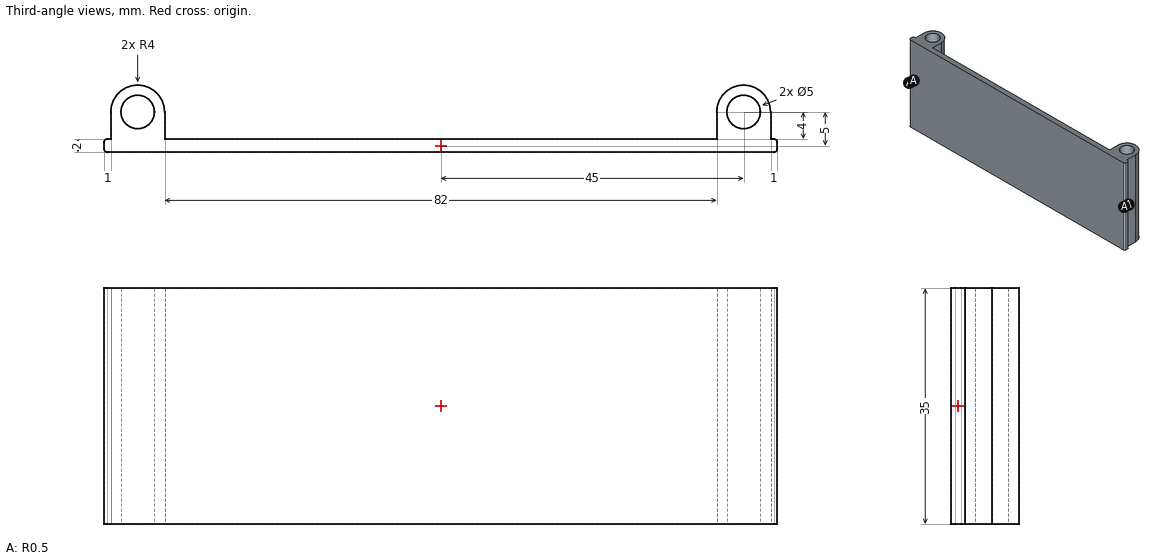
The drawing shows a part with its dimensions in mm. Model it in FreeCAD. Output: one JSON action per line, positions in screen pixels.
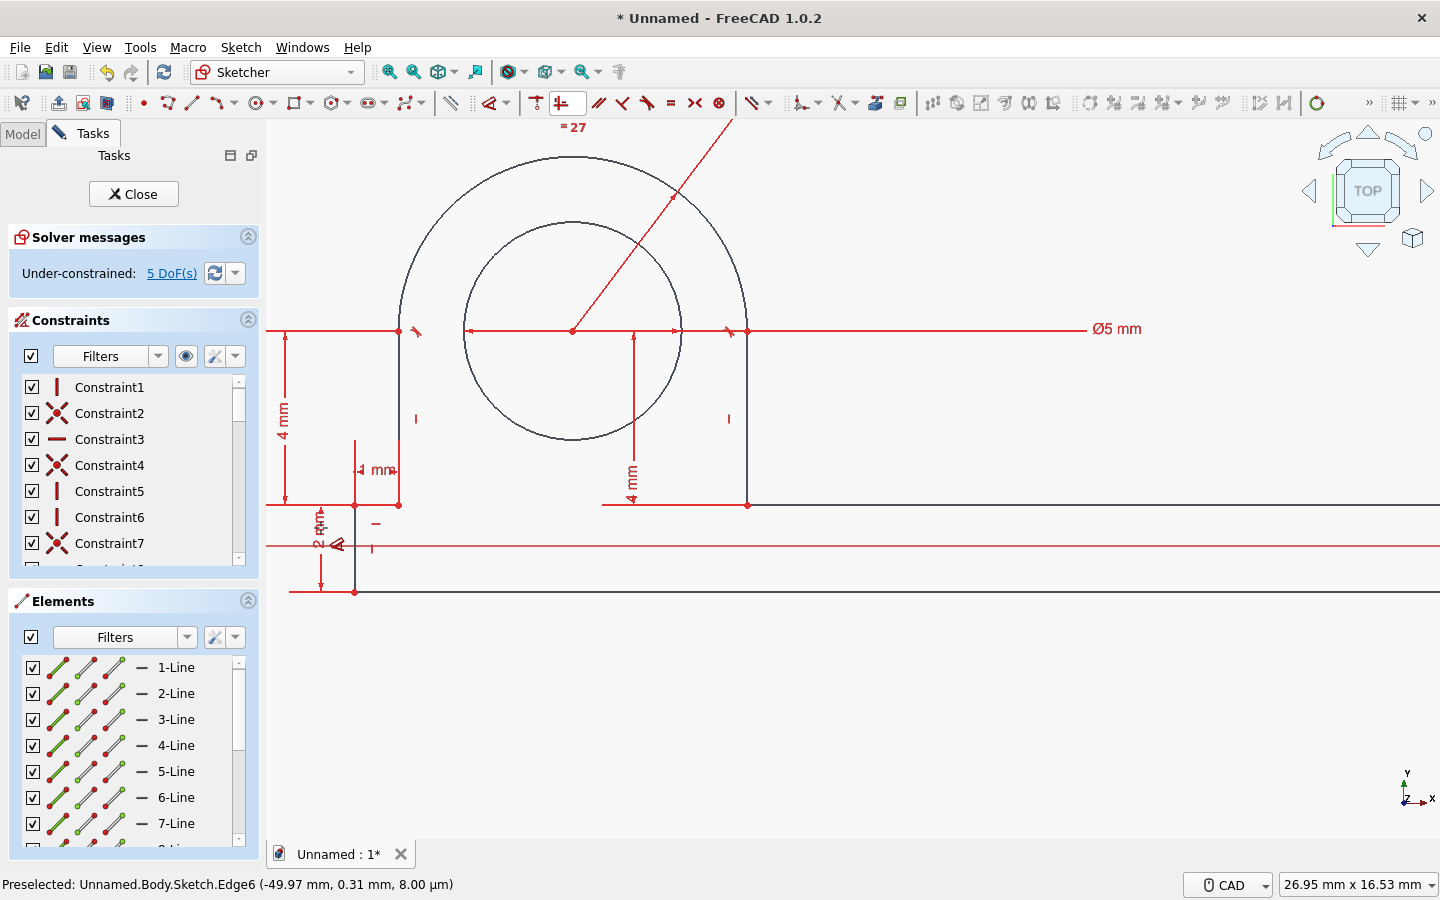
{"action": "scroll", "coordinate": [438, 500], "scroll_direction": "down", "scroll_amount": 9}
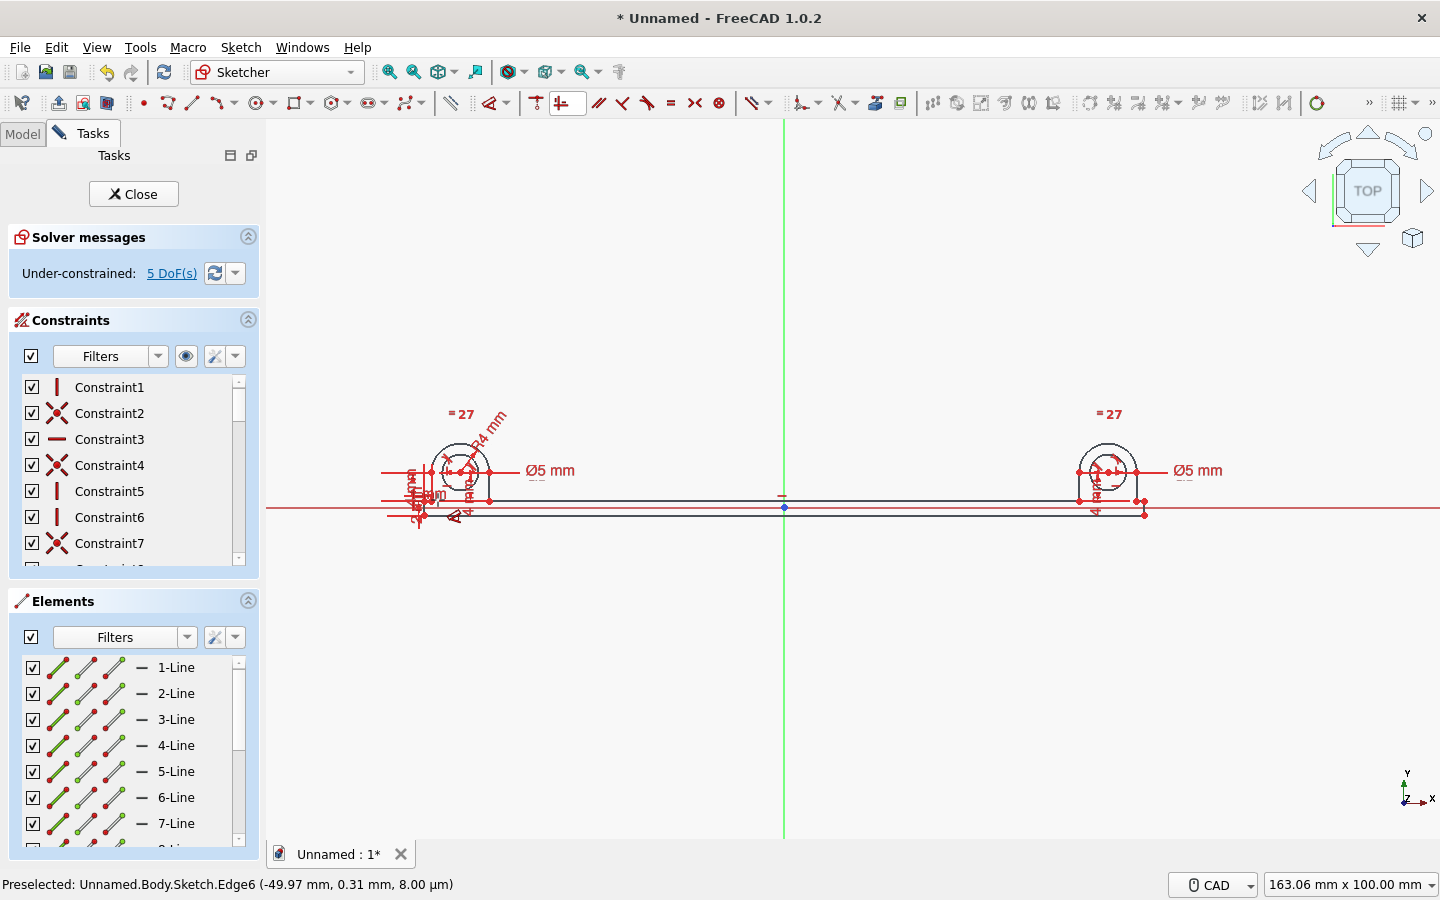
{"action": "scroll", "coordinate": [1144, 511], "scroll_direction": "up", "scroll_amount": 8}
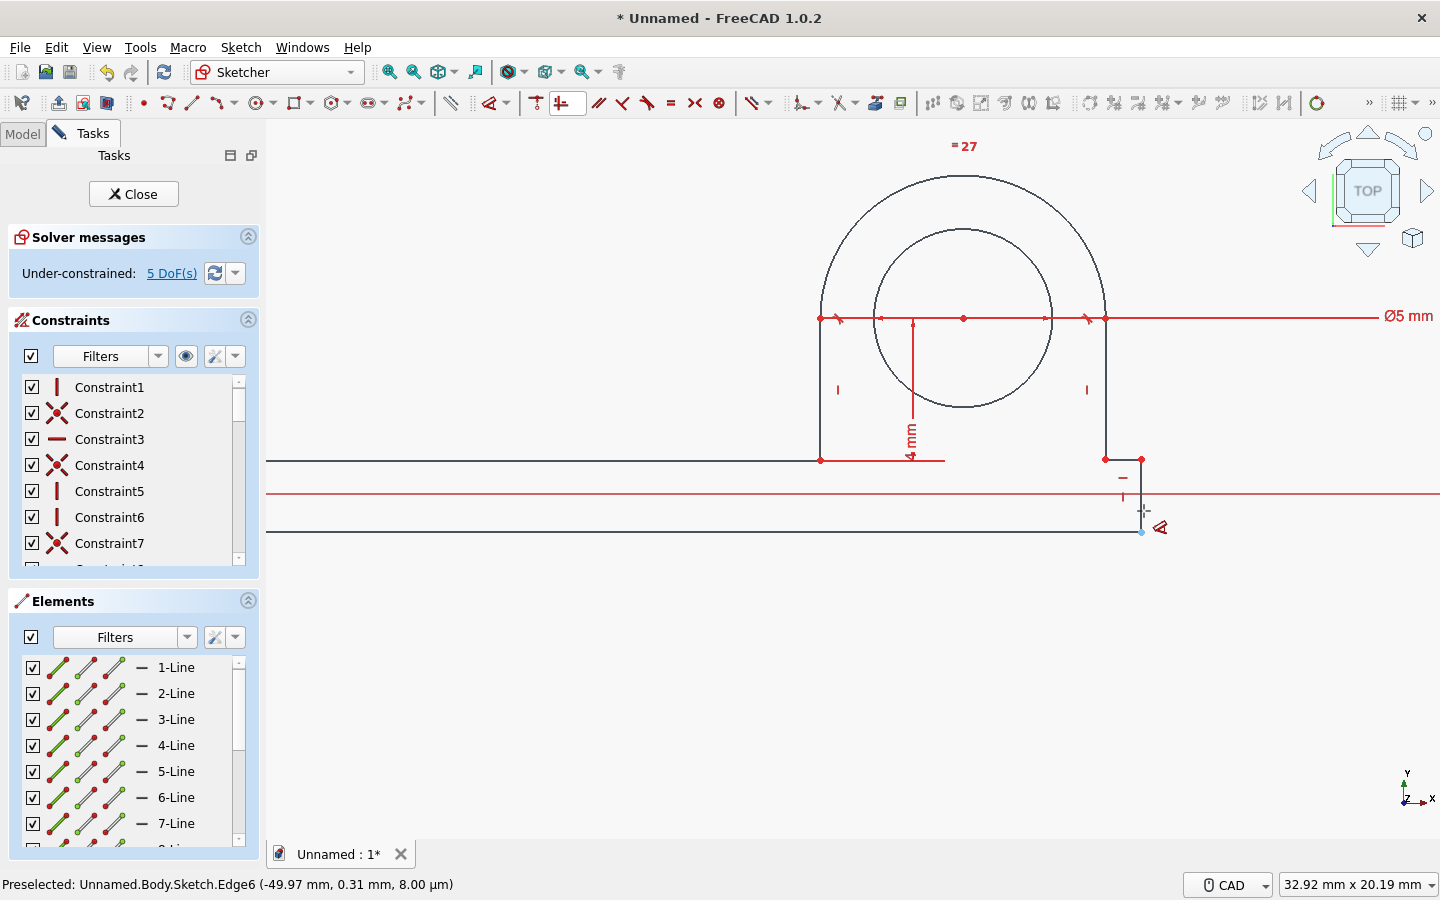
{"action": "left_click", "coordinate": [1141, 511]}
{"action": "left_click", "coordinate": [1175, 479]}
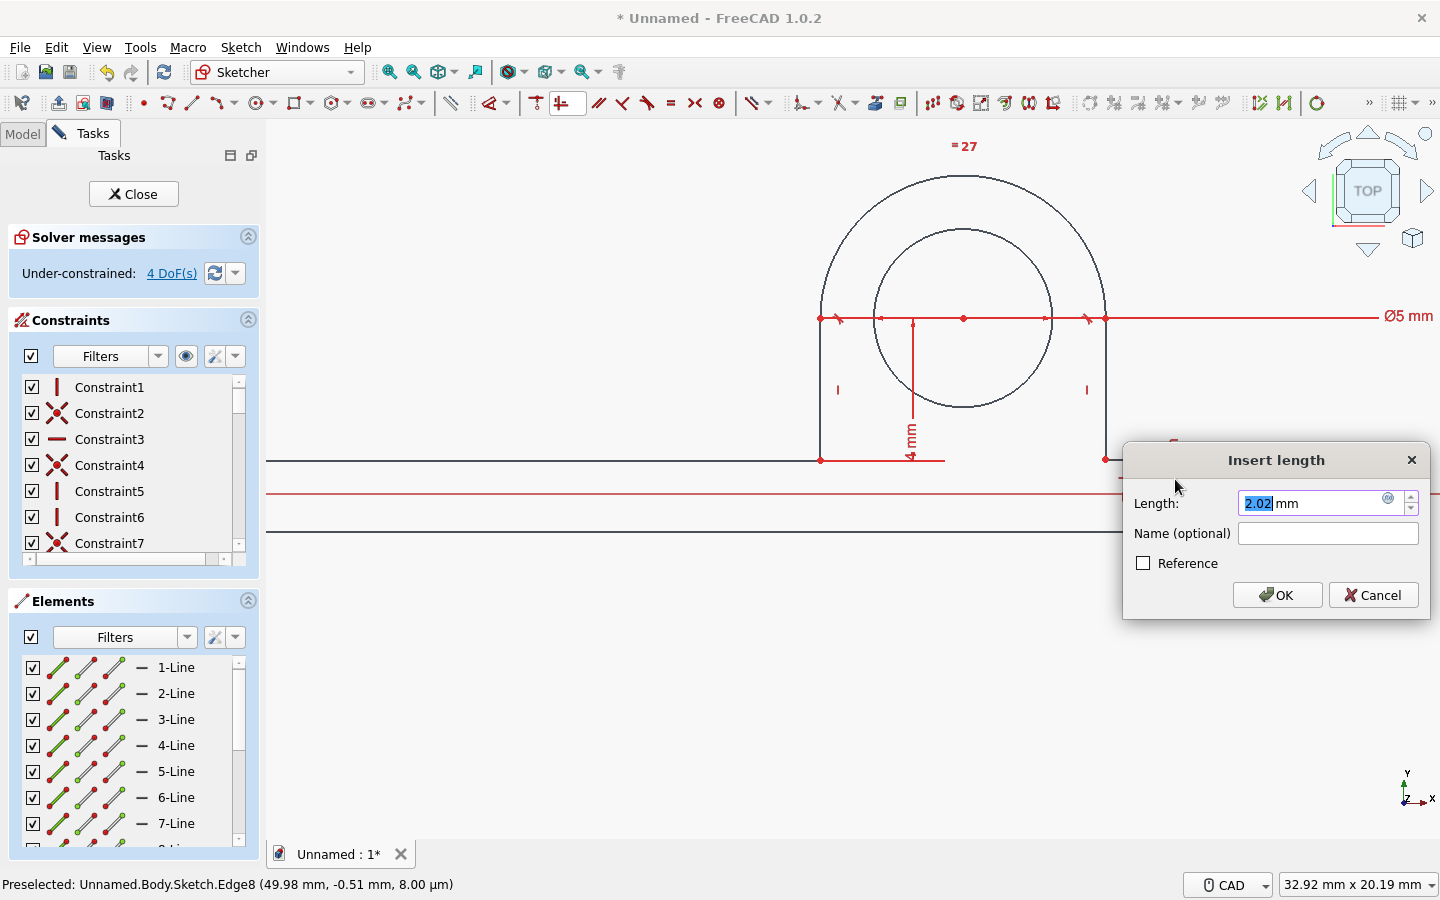
{"action": "type", "text": "2"}
{"action": "key", "text": "Return"}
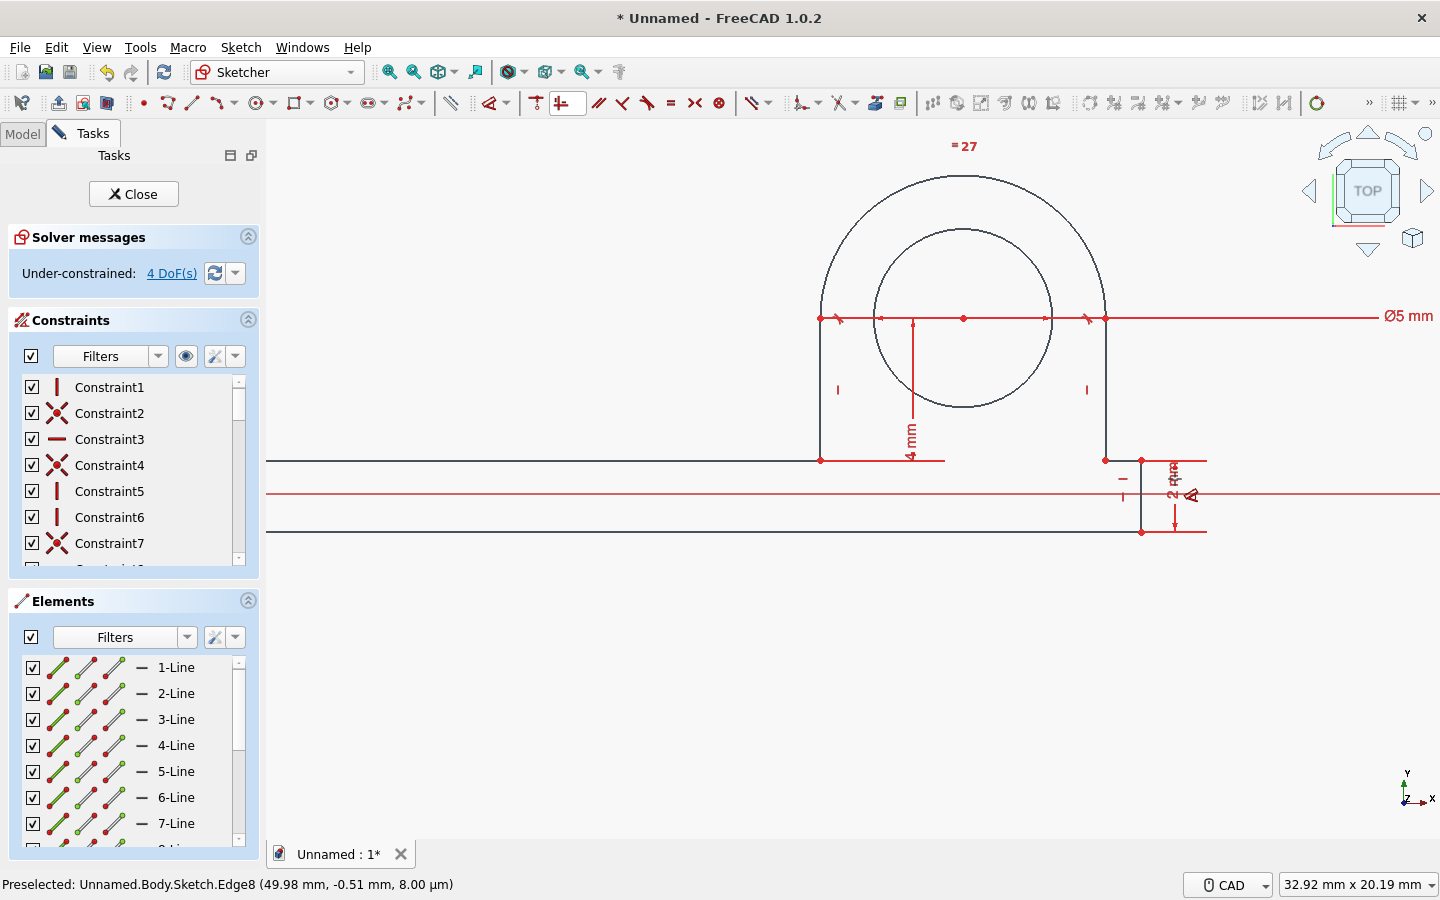
{"action": "scroll", "coordinate": [1131, 461], "scroll_direction": "up", "scroll_amount": 2}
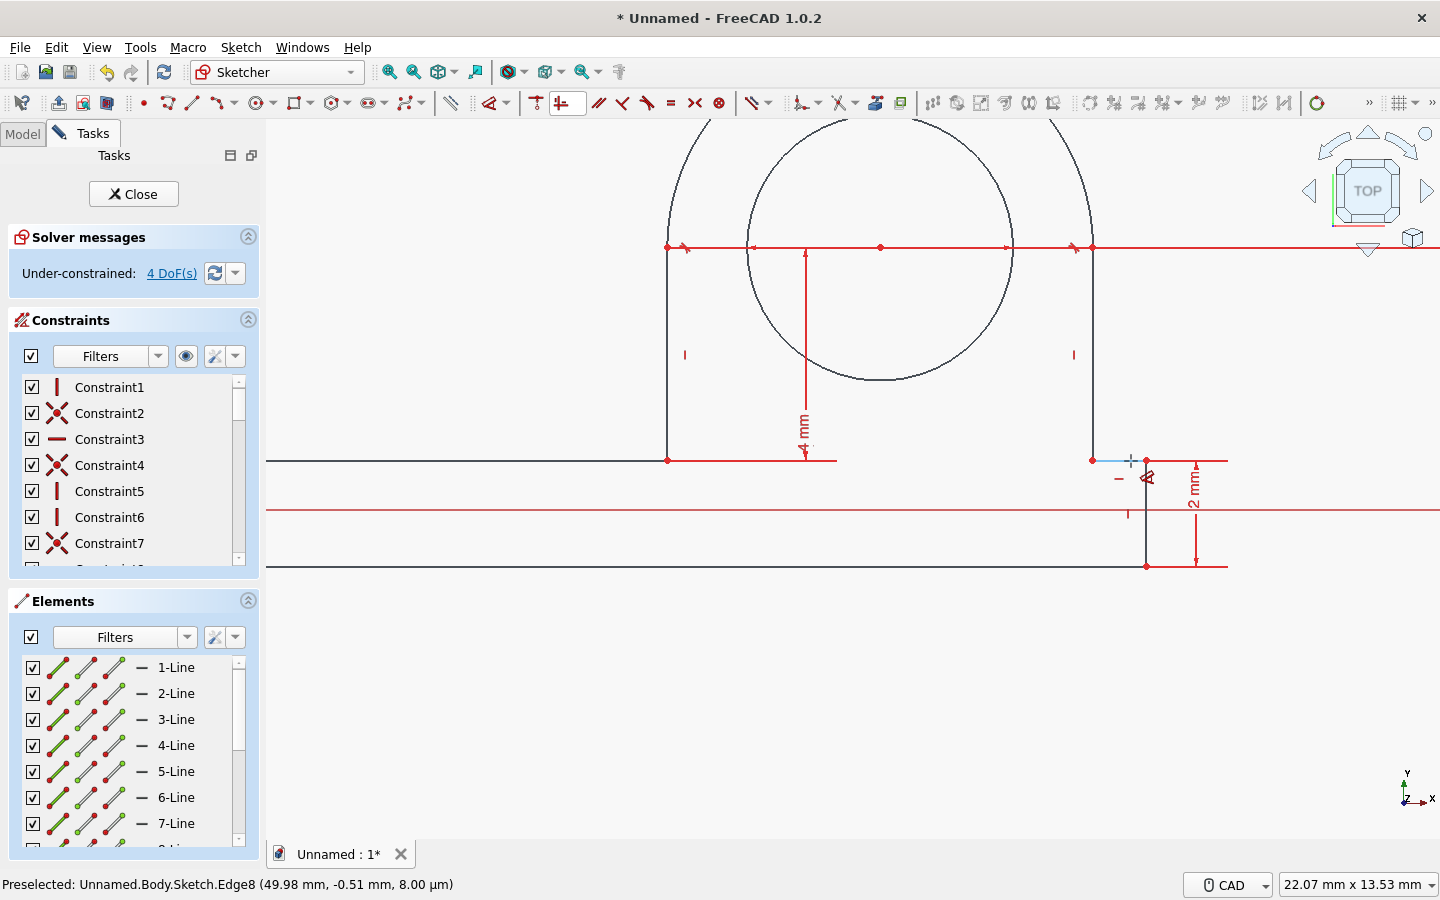
{"action": "left_click", "coordinate": [1130, 461]}
{"action": "left_click", "coordinate": [1119, 495]}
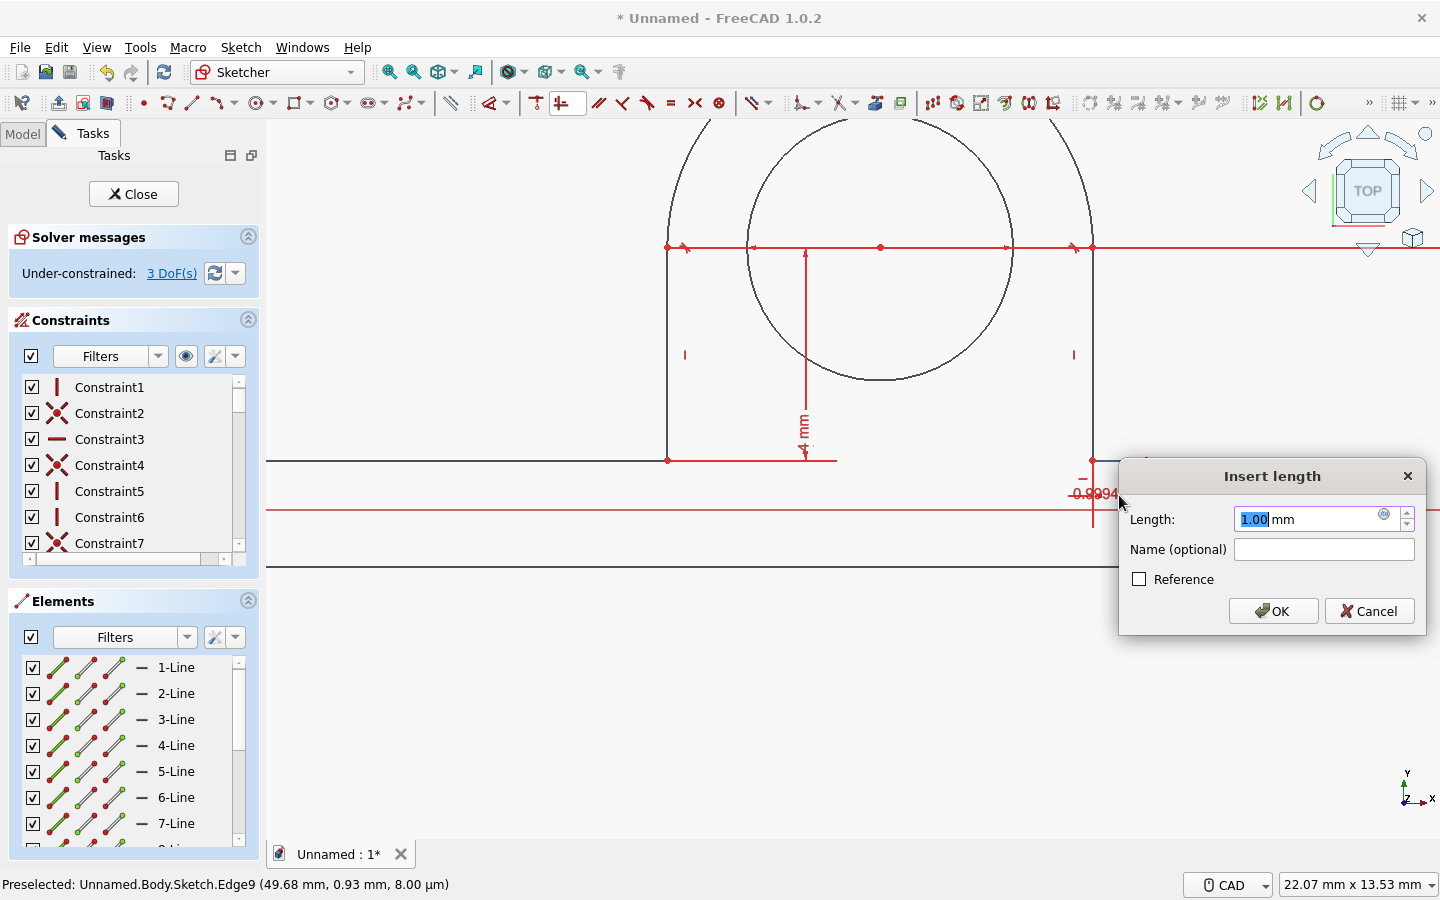
{"action": "type", "text": "1"}
{"action": "key", "text": "Return"}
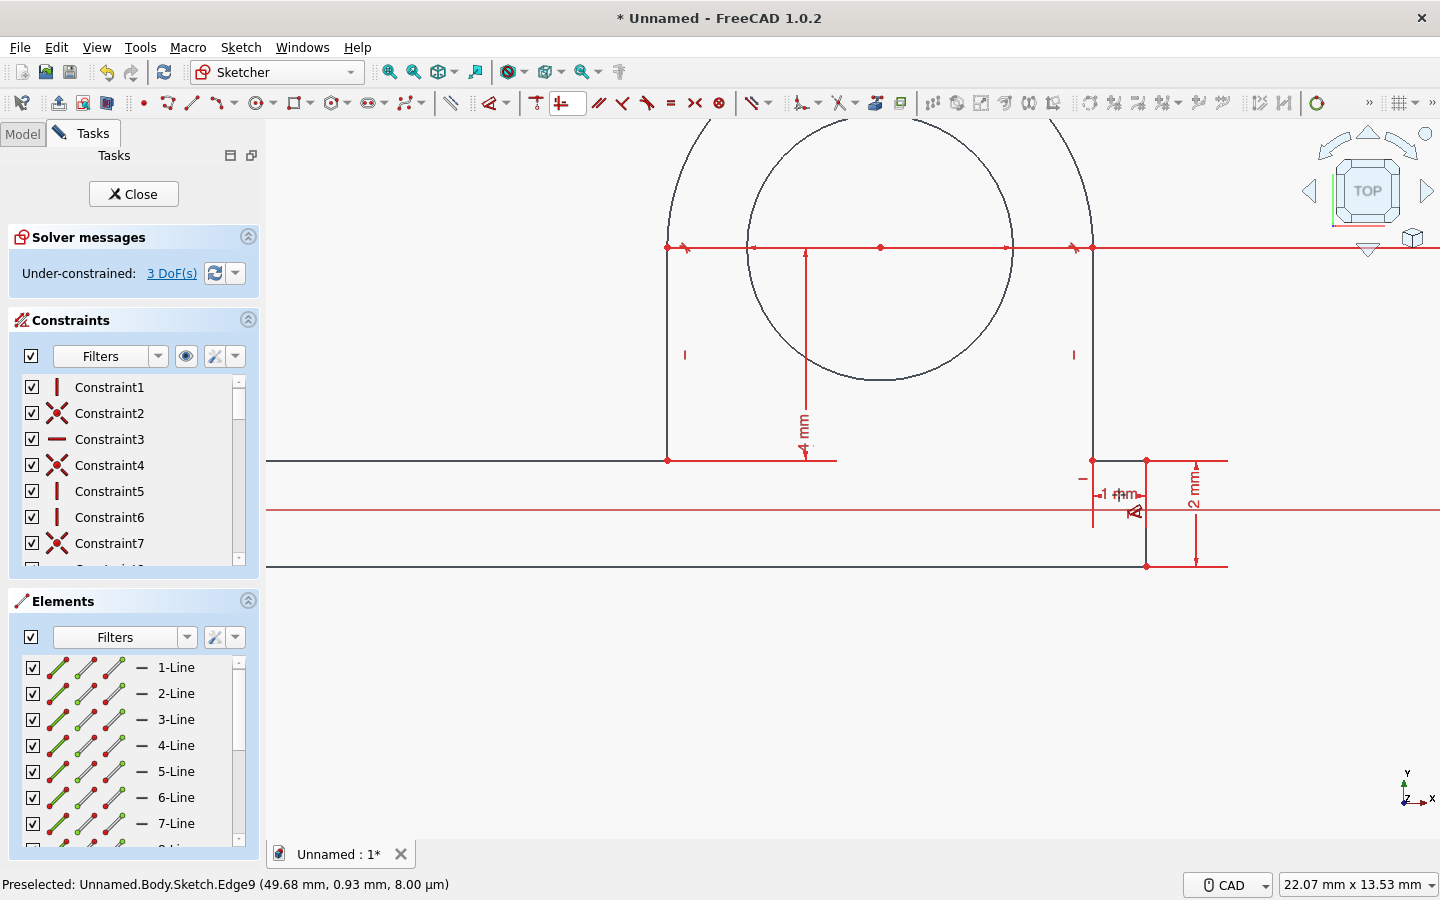
{"action": "scroll", "coordinate": [1144, 507], "scroll_direction": "down", "scroll_amount": 10}